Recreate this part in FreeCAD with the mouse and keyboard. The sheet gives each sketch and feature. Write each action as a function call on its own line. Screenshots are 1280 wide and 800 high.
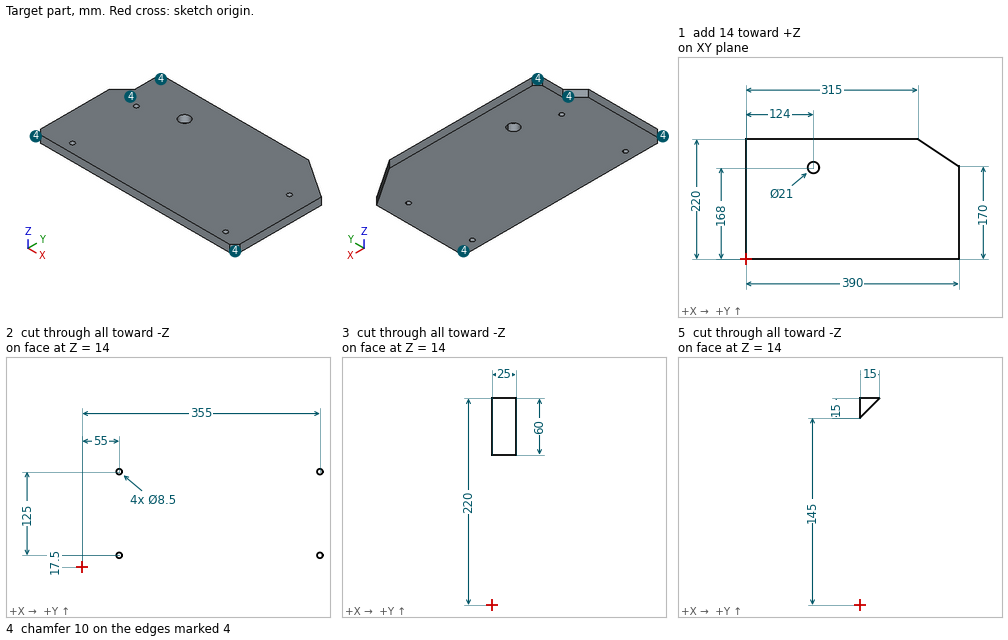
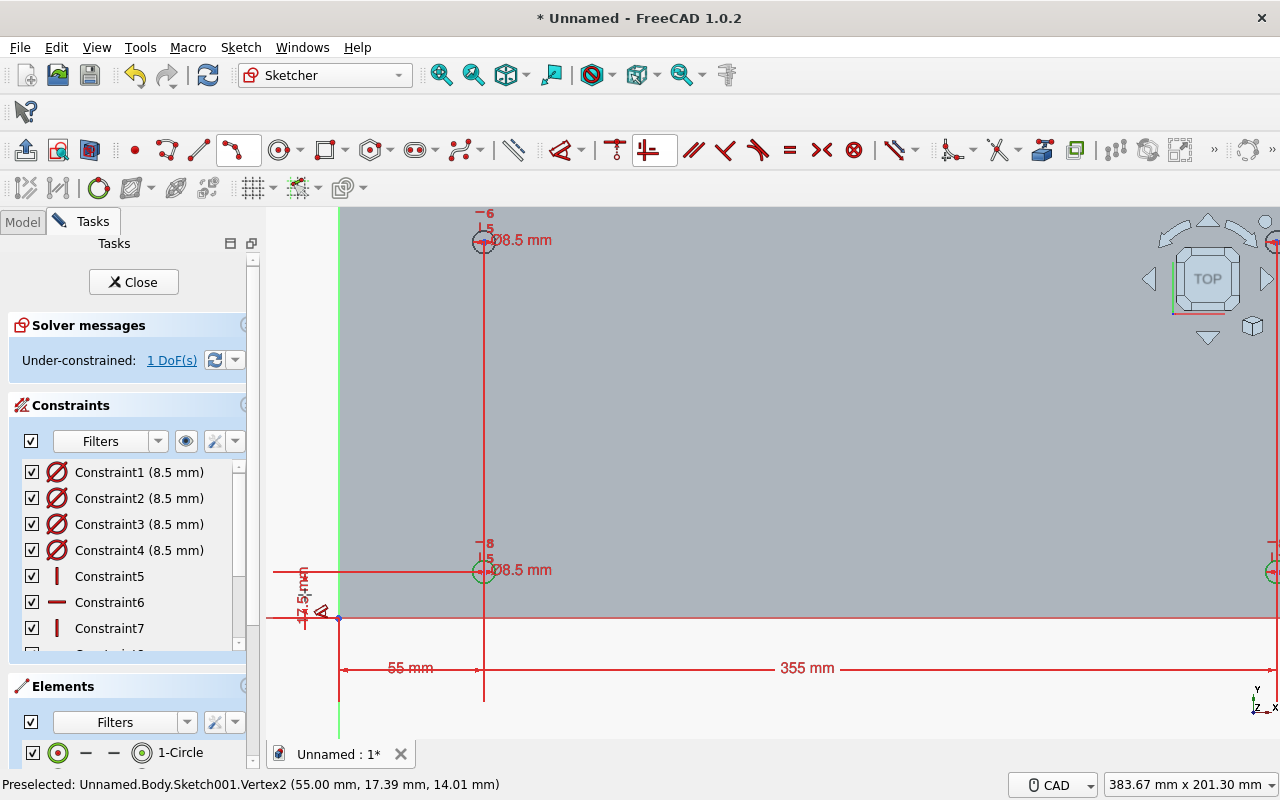
click(484, 242)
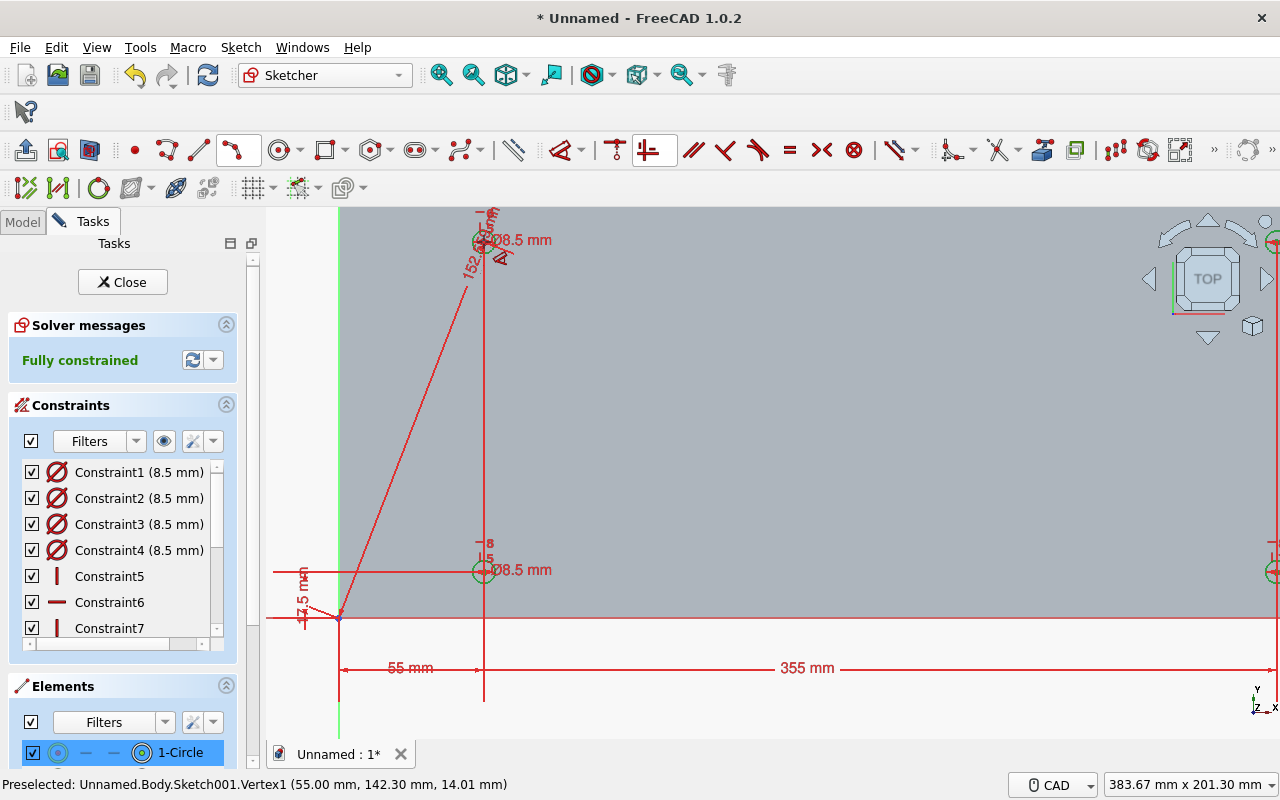
click(484, 572)
click(450, 407)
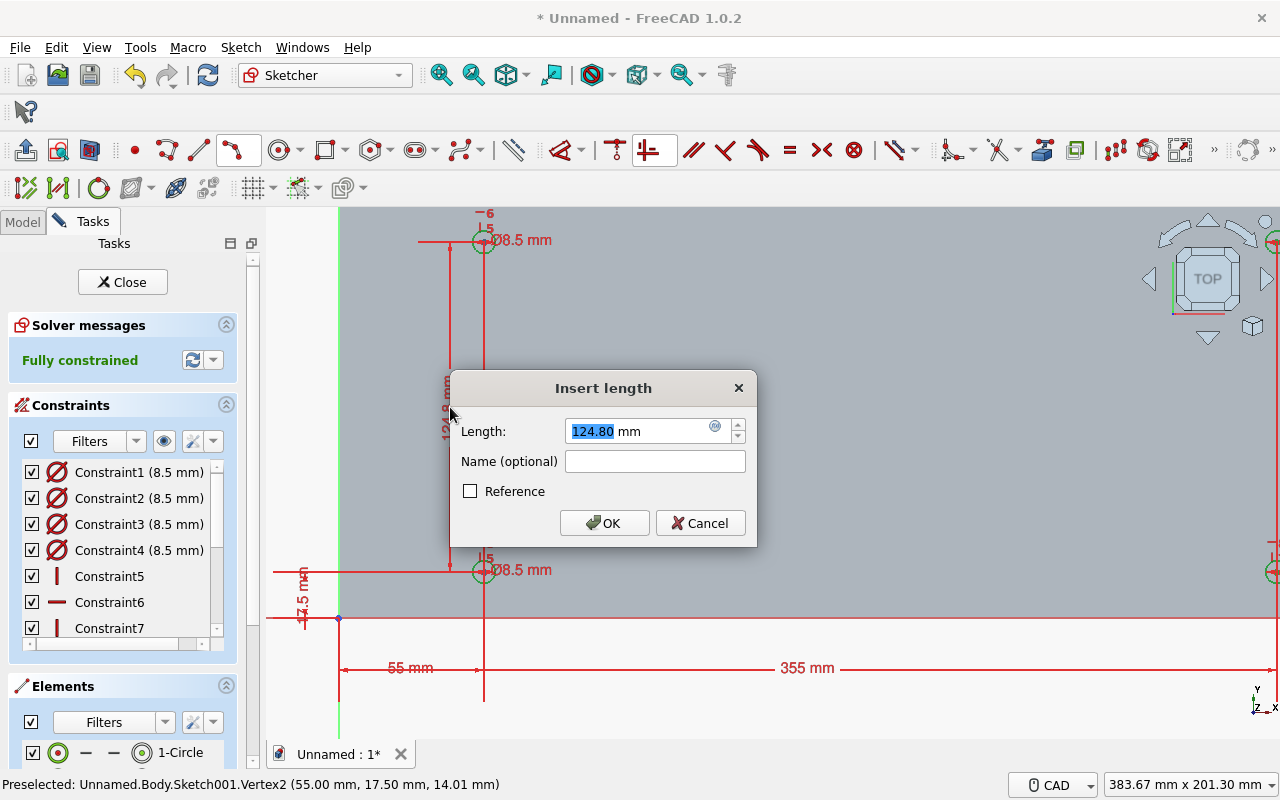
text(125)
key(Return)
key(Escape)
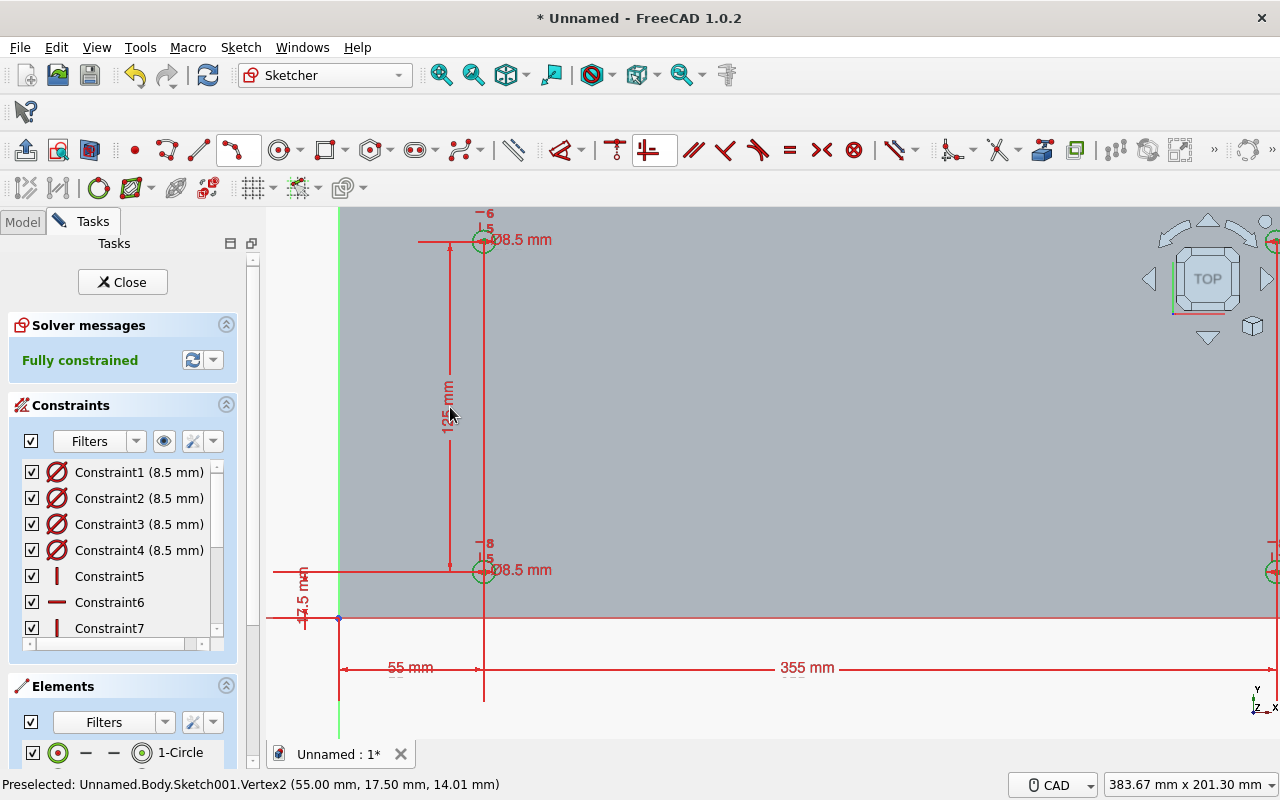
click(123, 282)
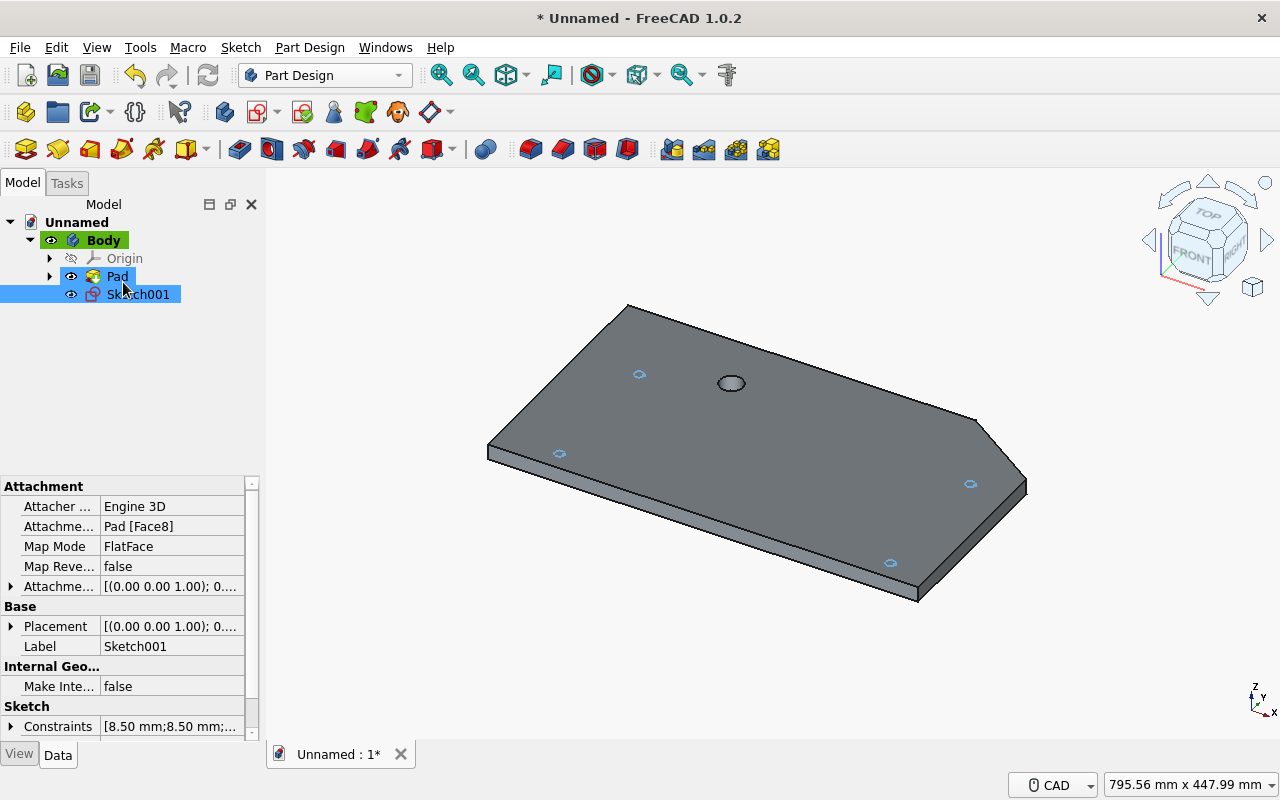
click(240, 150)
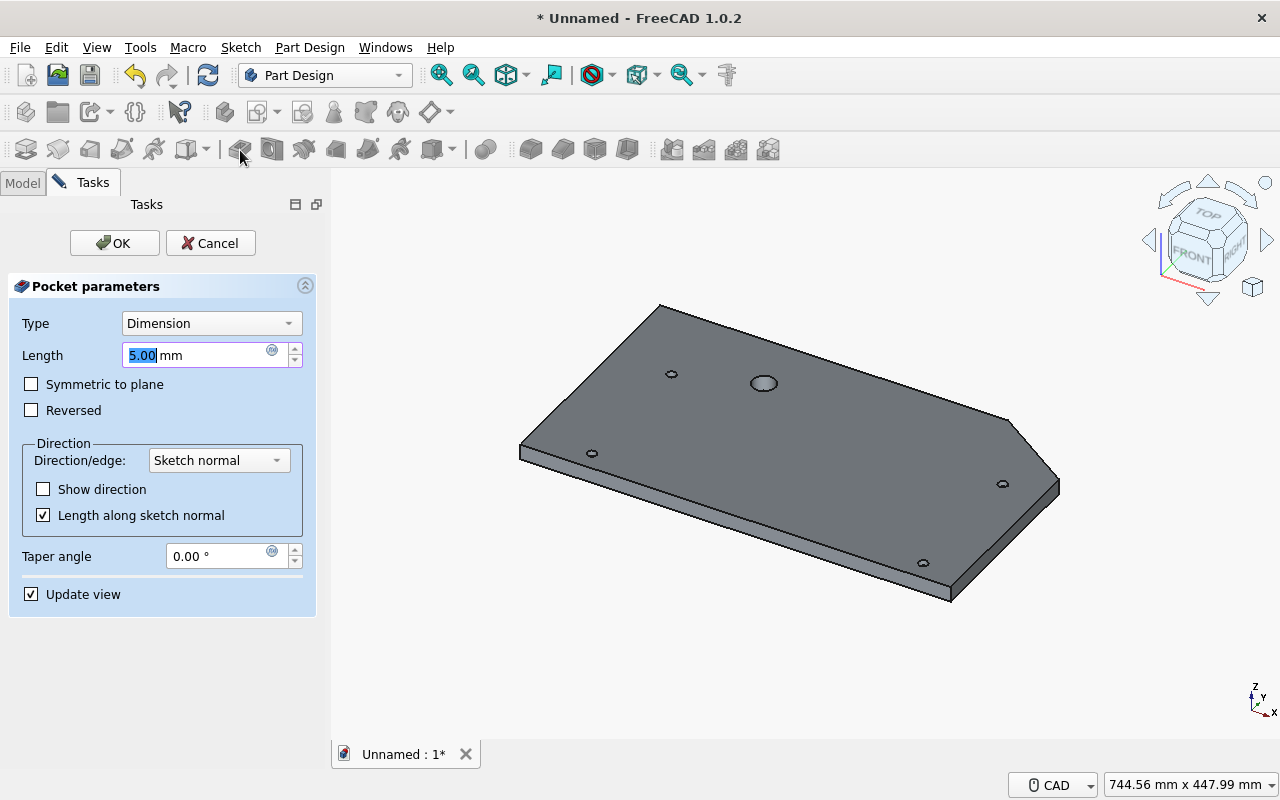
click(212, 324)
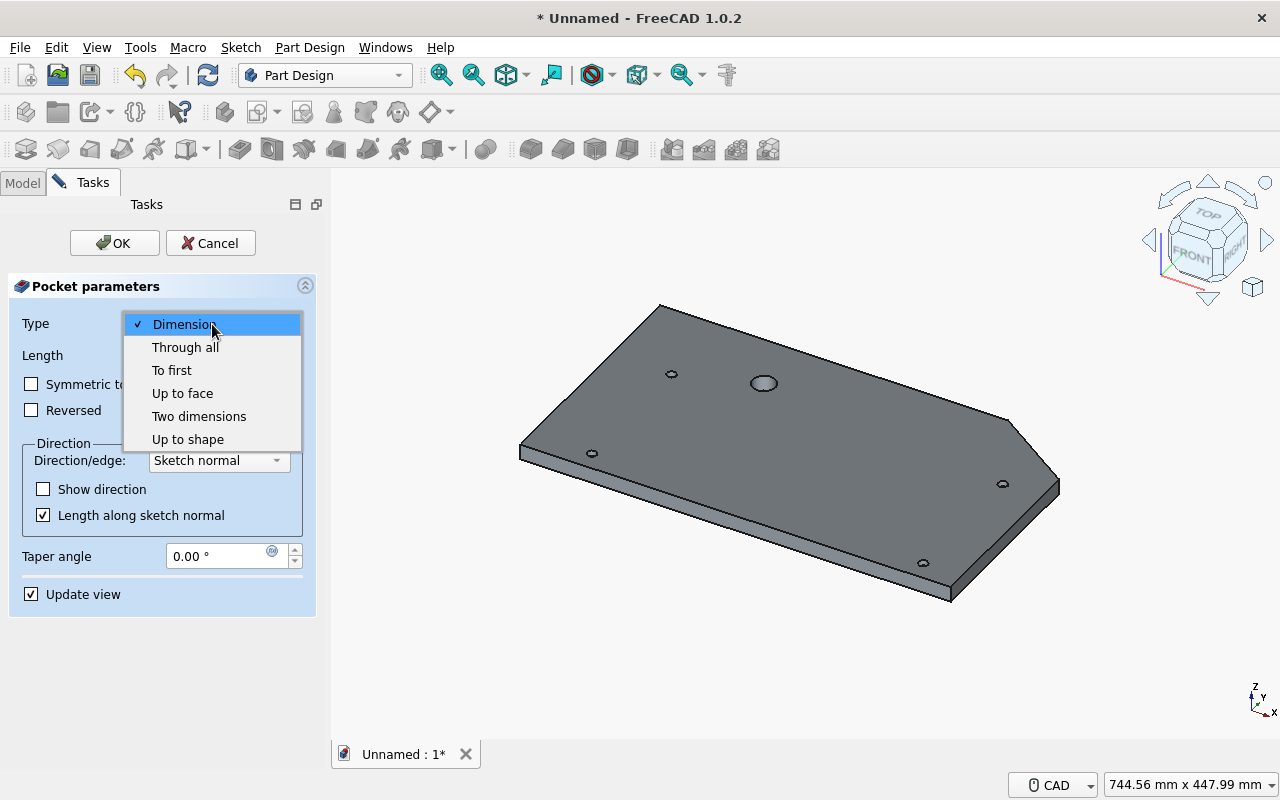
click(212, 348)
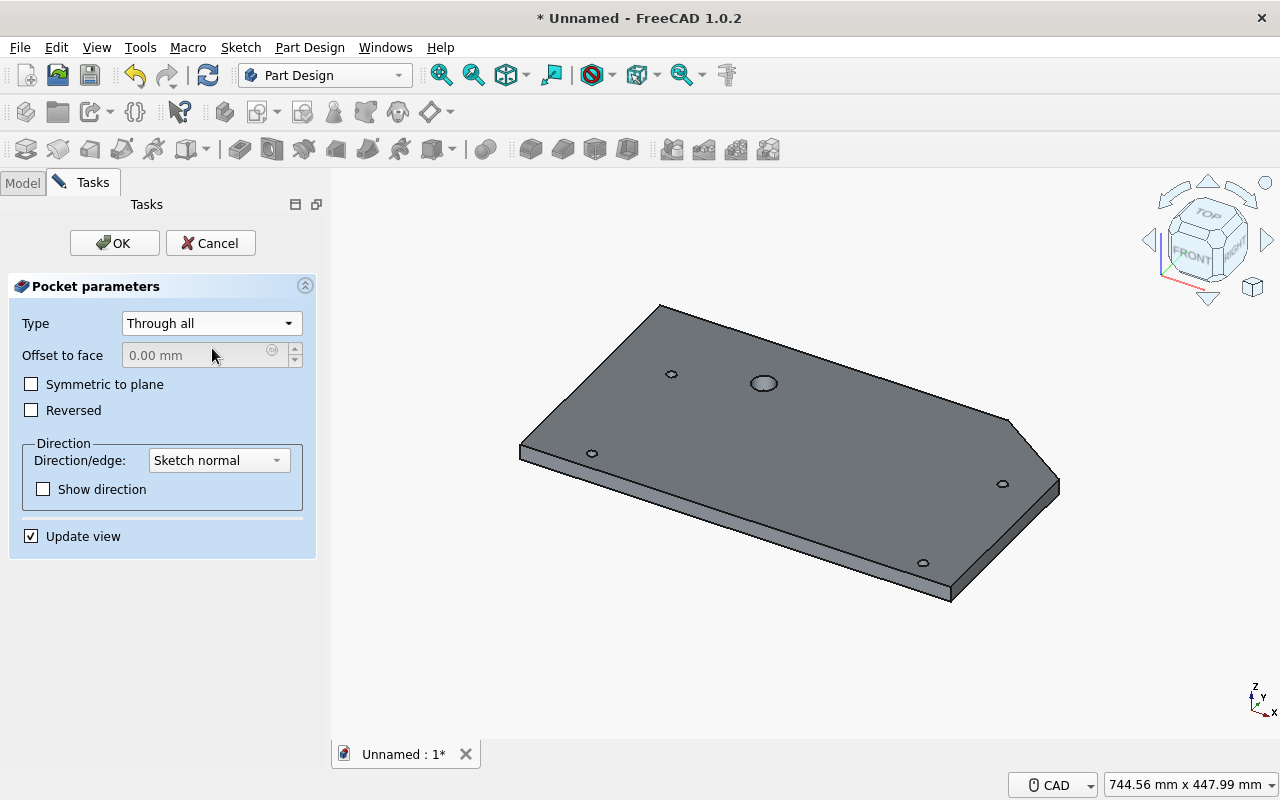
click(115, 243)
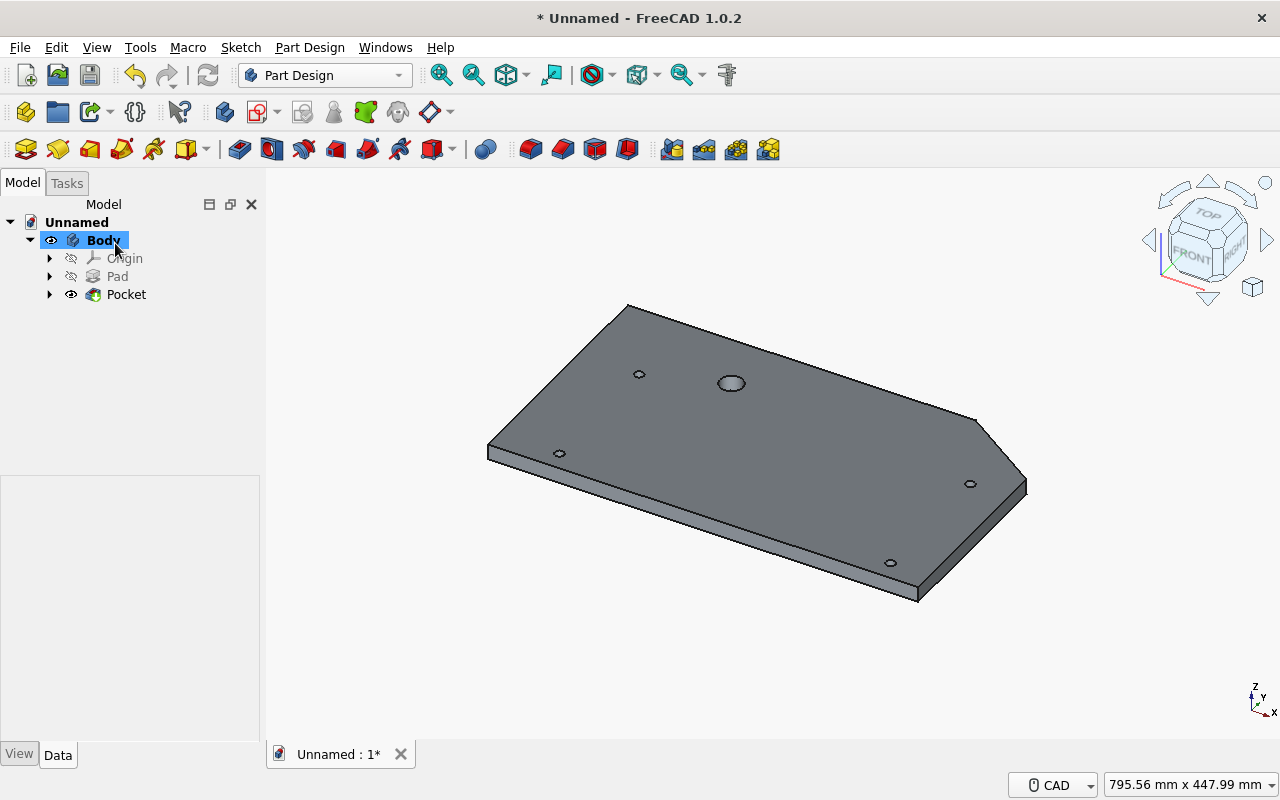
click(834, 466)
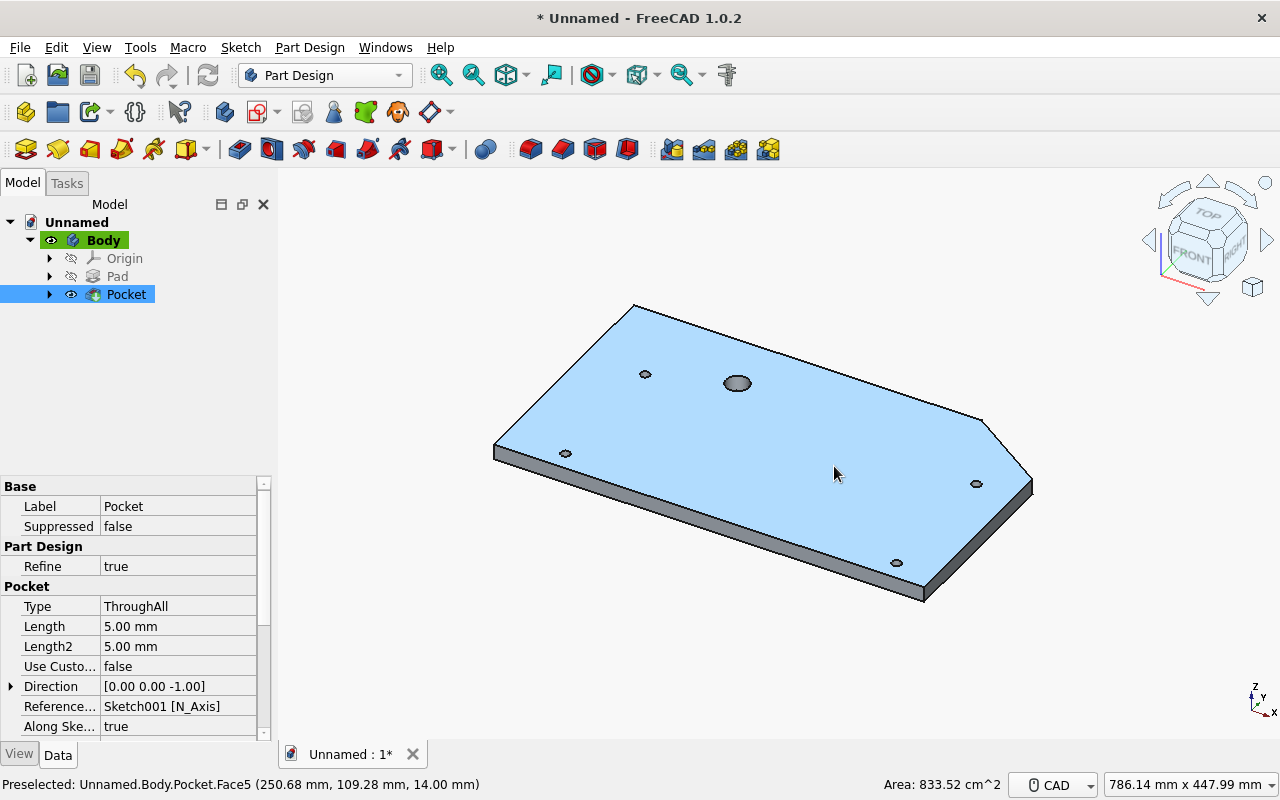
click(258, 112)